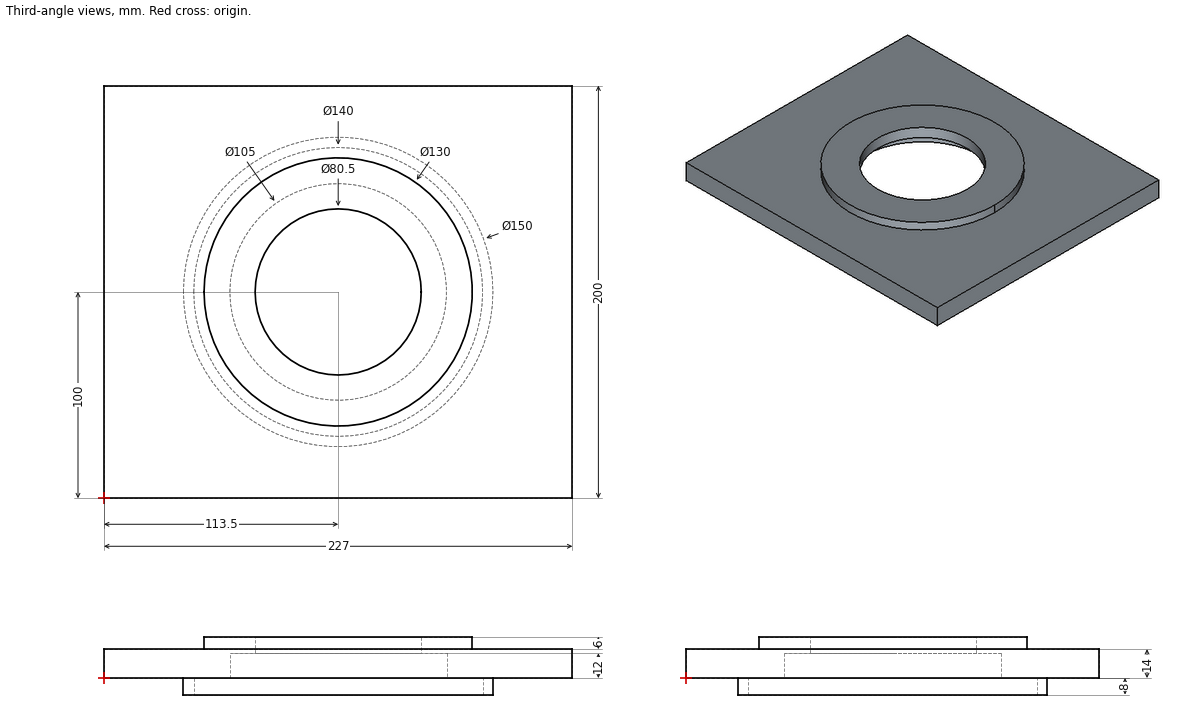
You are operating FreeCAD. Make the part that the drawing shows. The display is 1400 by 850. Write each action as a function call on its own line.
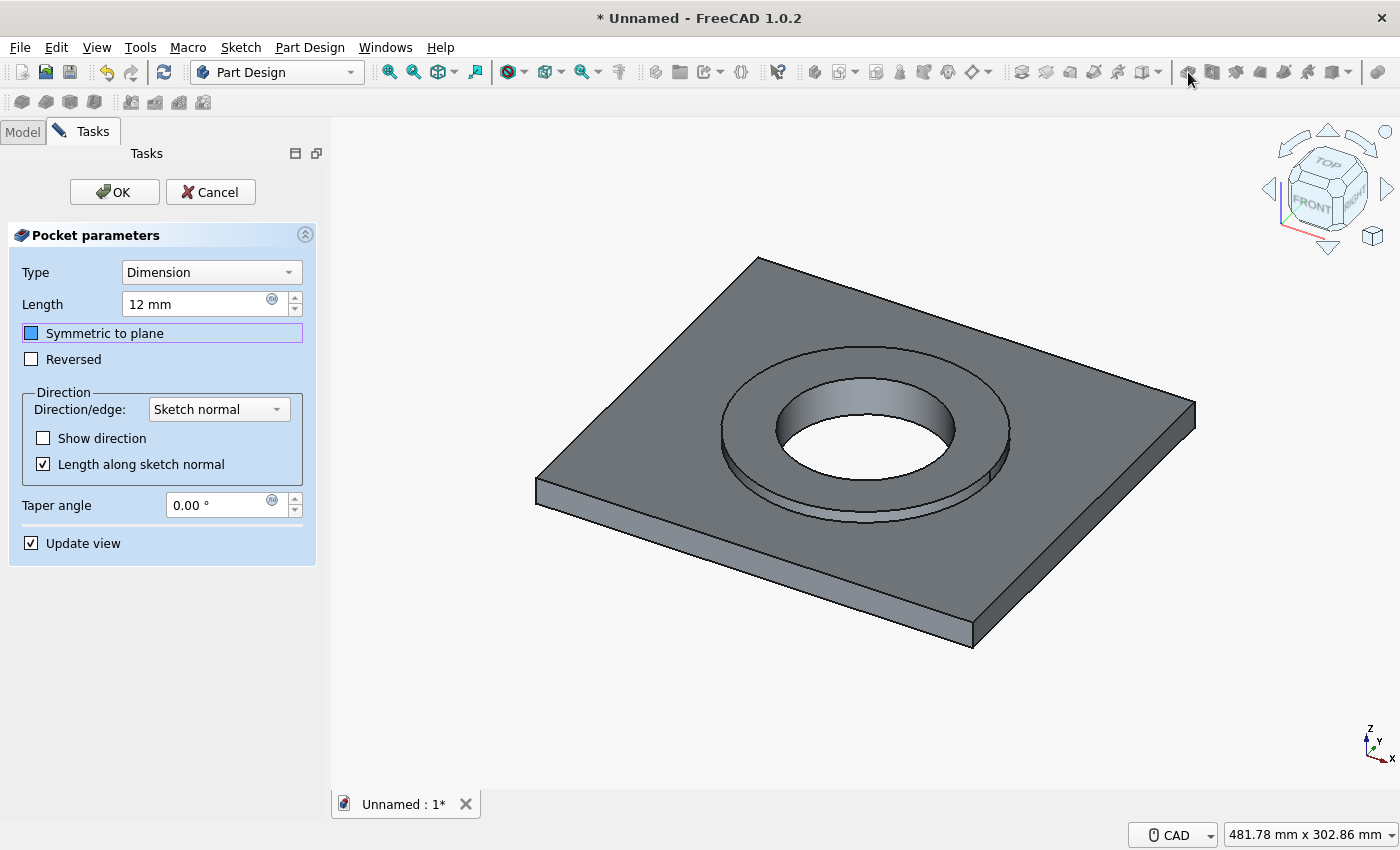
click(30, 359)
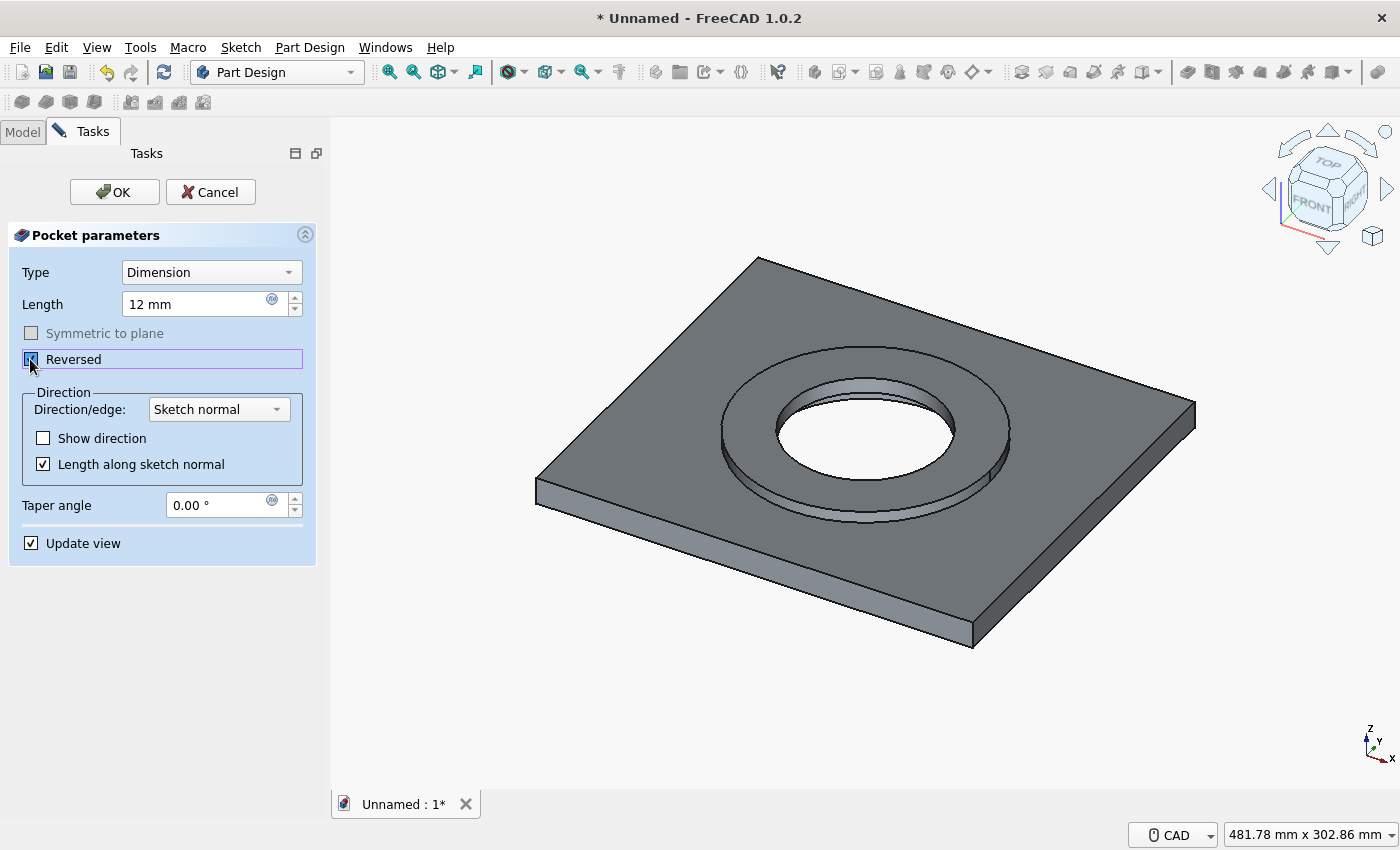
click(115, 192)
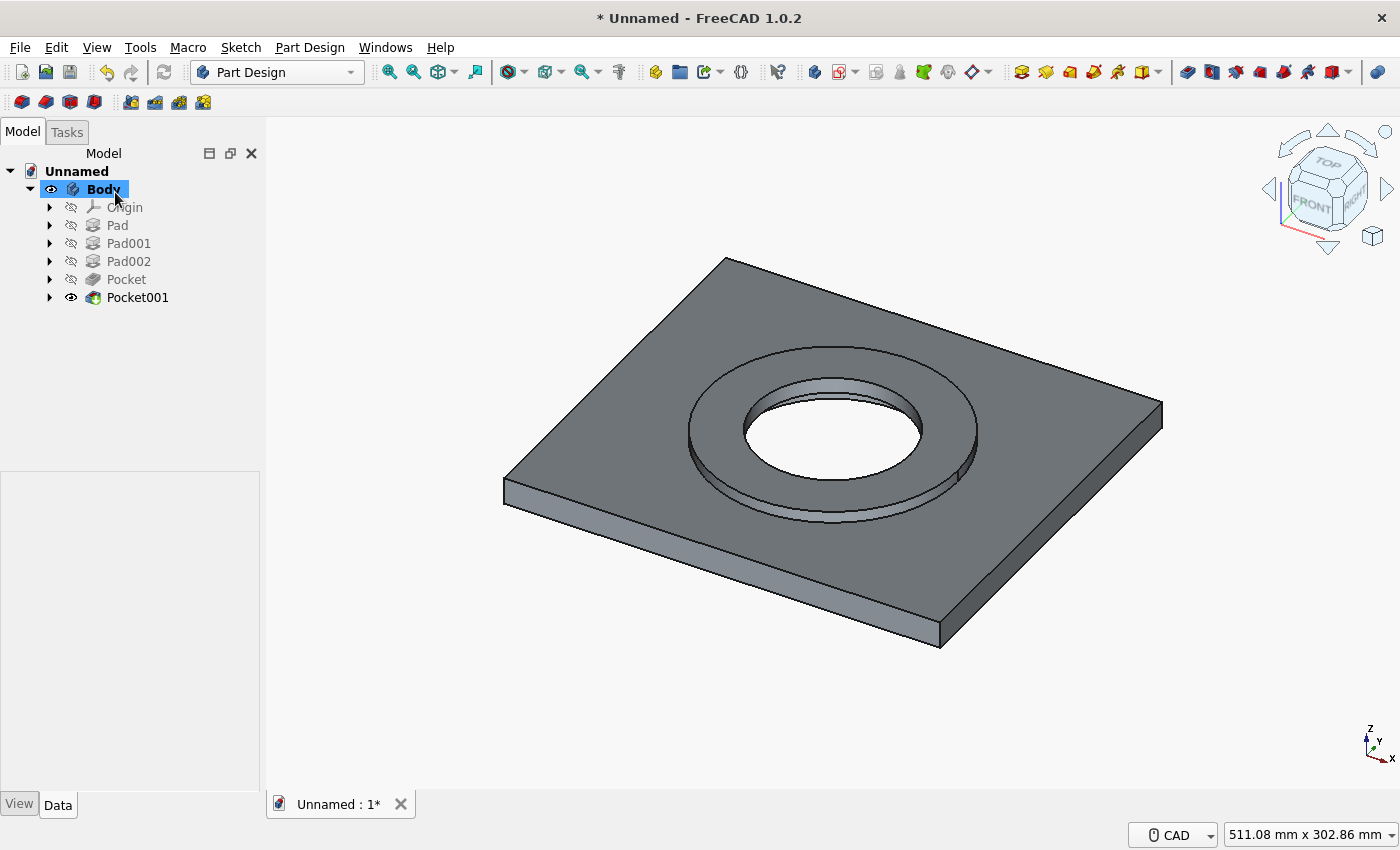
key(0)